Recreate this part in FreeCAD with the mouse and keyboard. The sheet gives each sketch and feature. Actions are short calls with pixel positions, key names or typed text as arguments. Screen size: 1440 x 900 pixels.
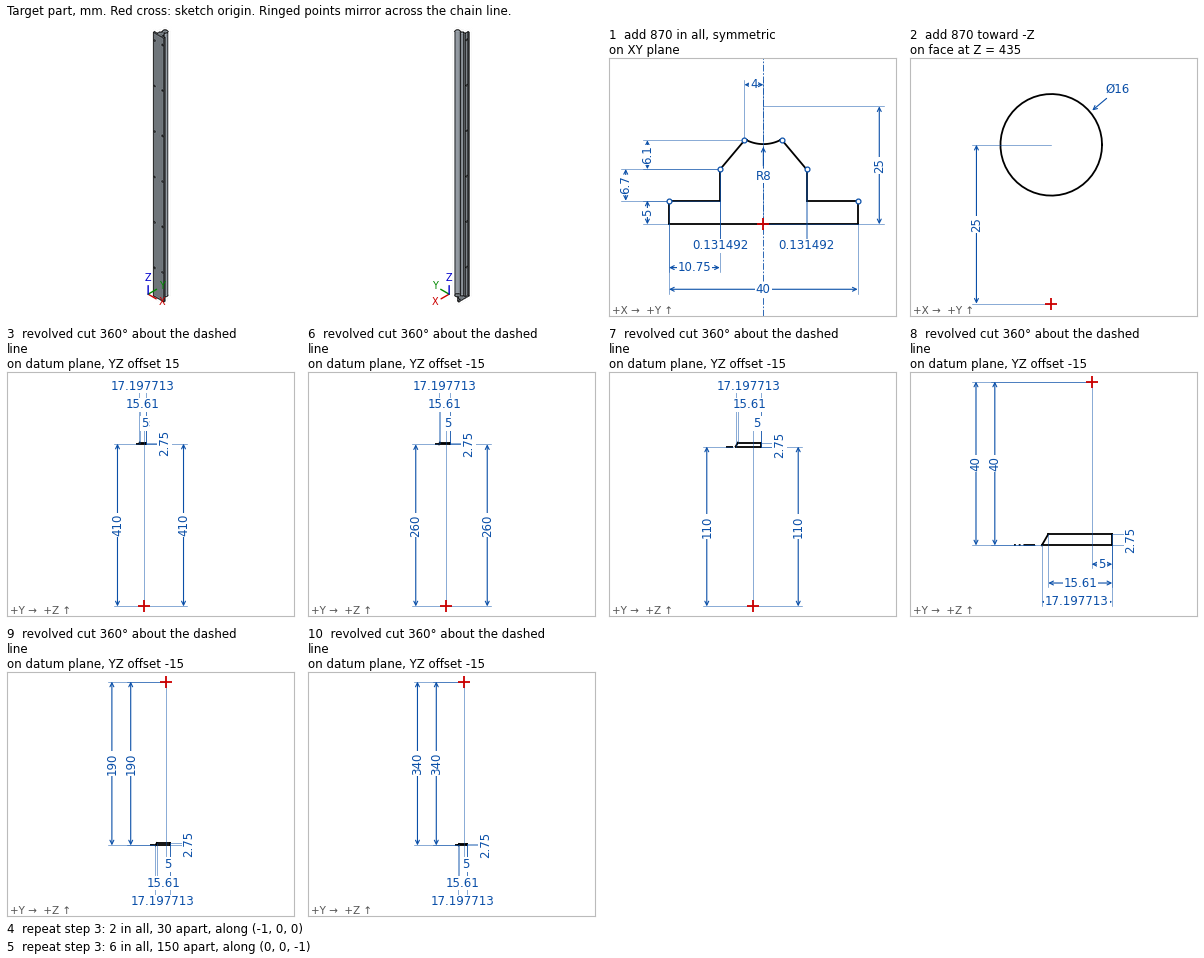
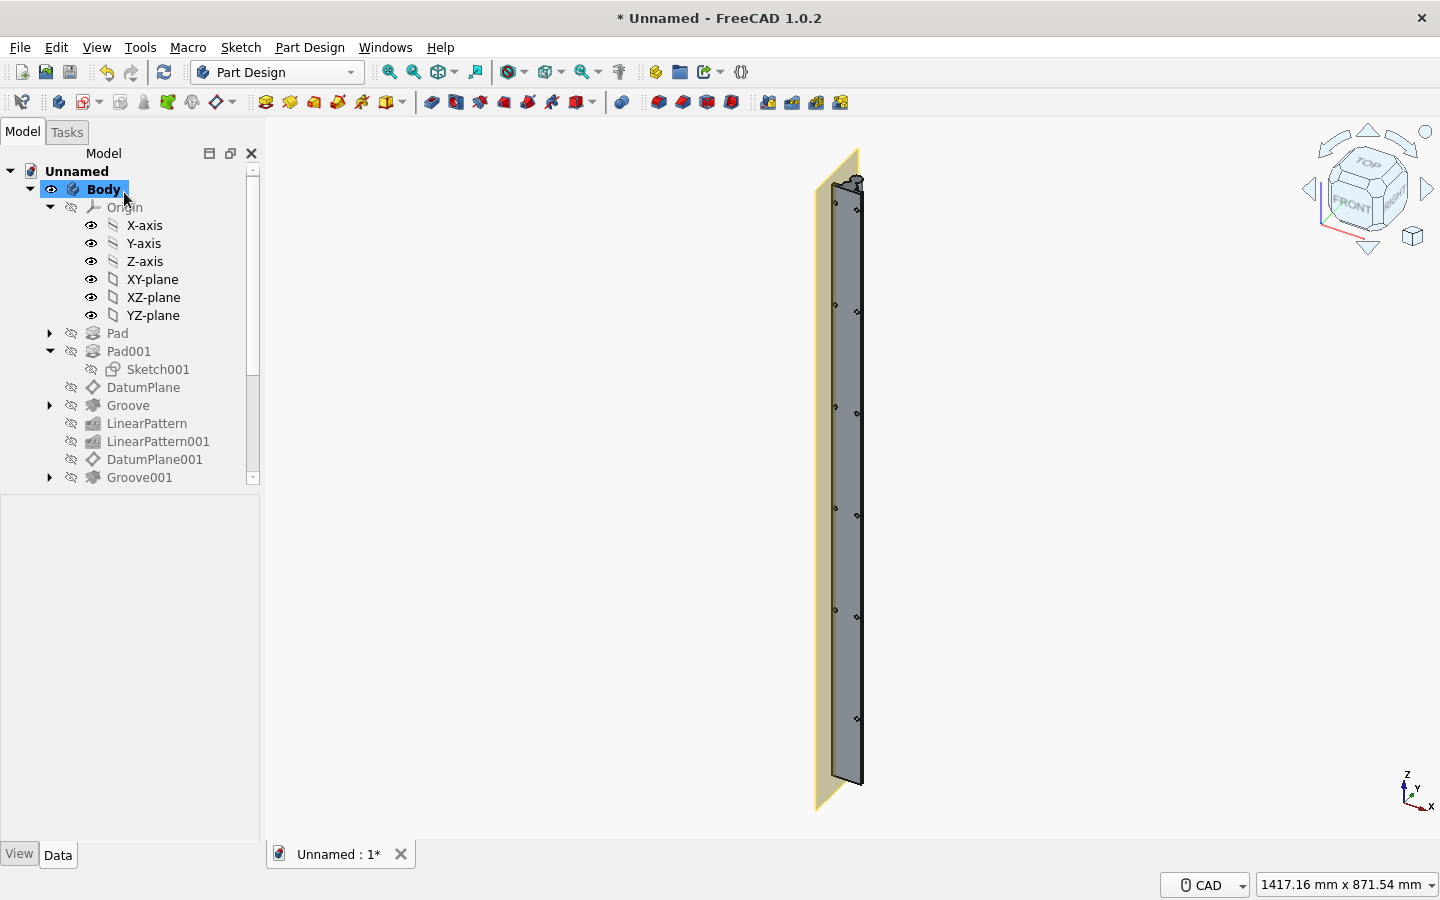
scroll(100, 329, down, 3)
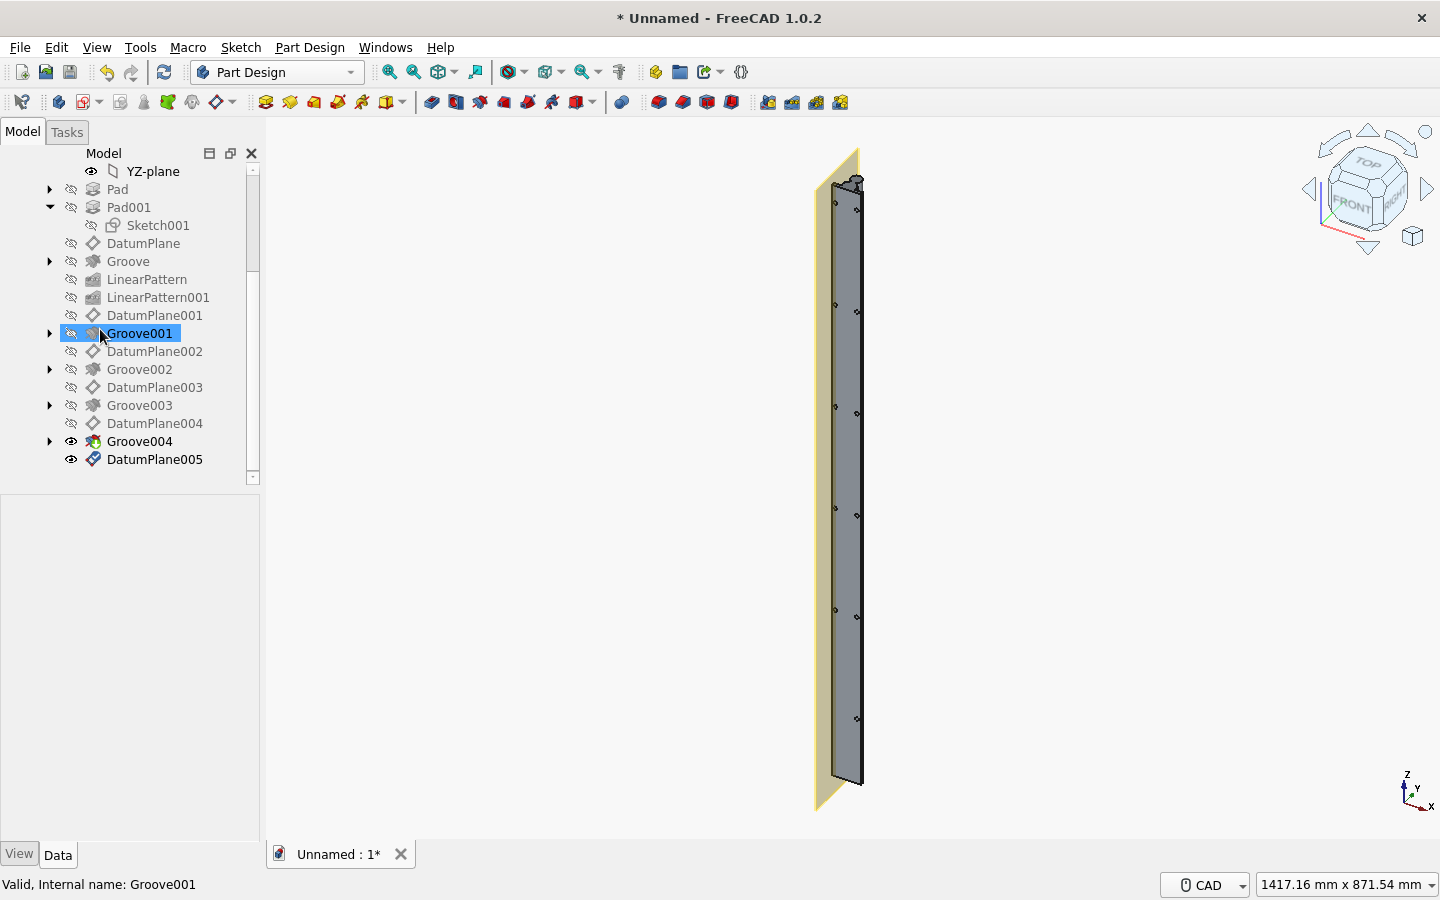
click(116, 459)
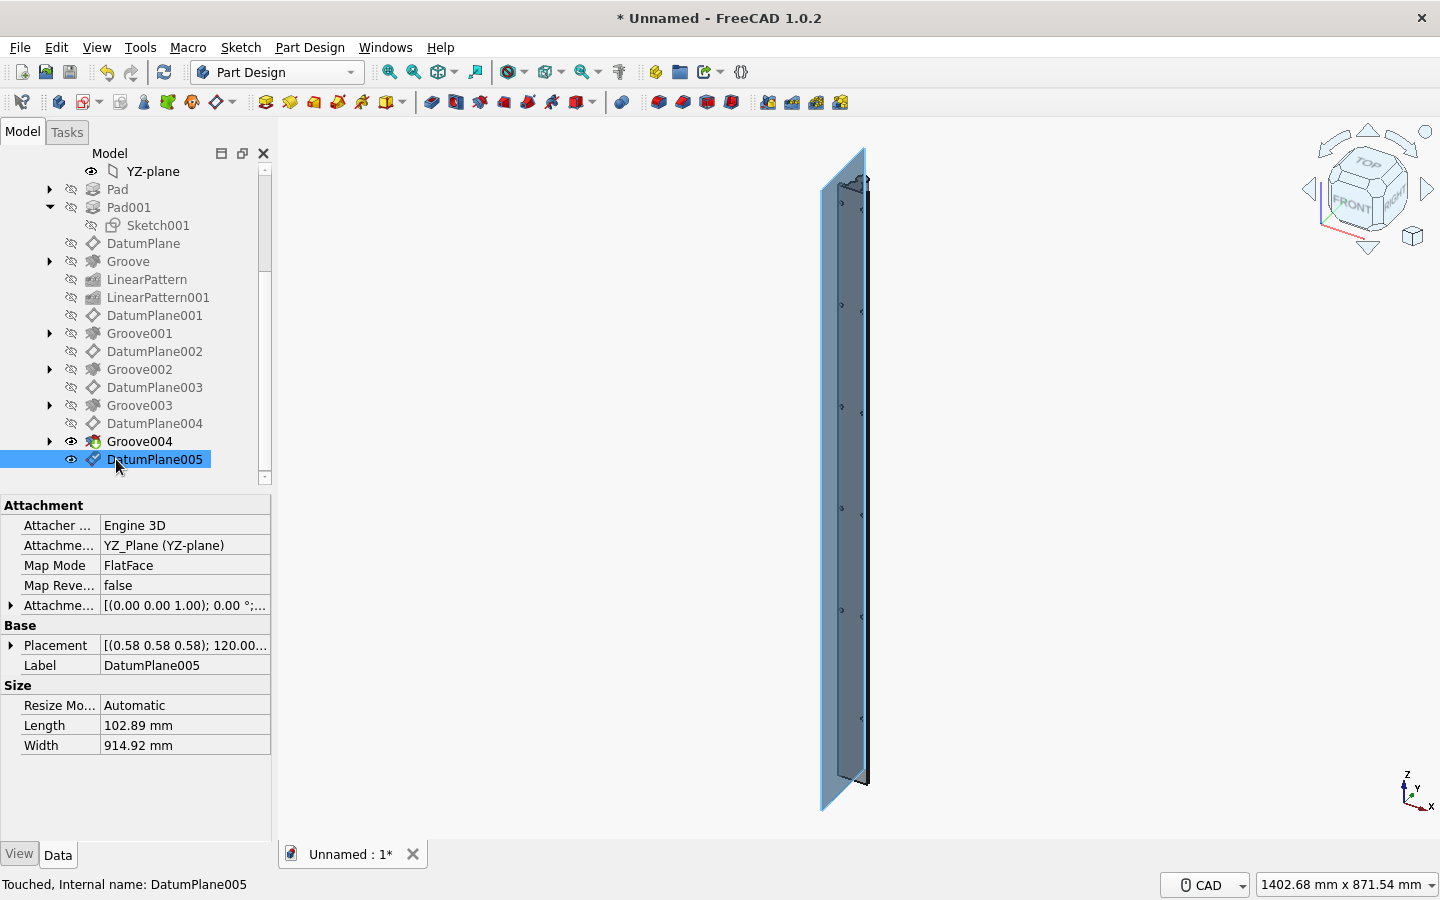
click(84, 102)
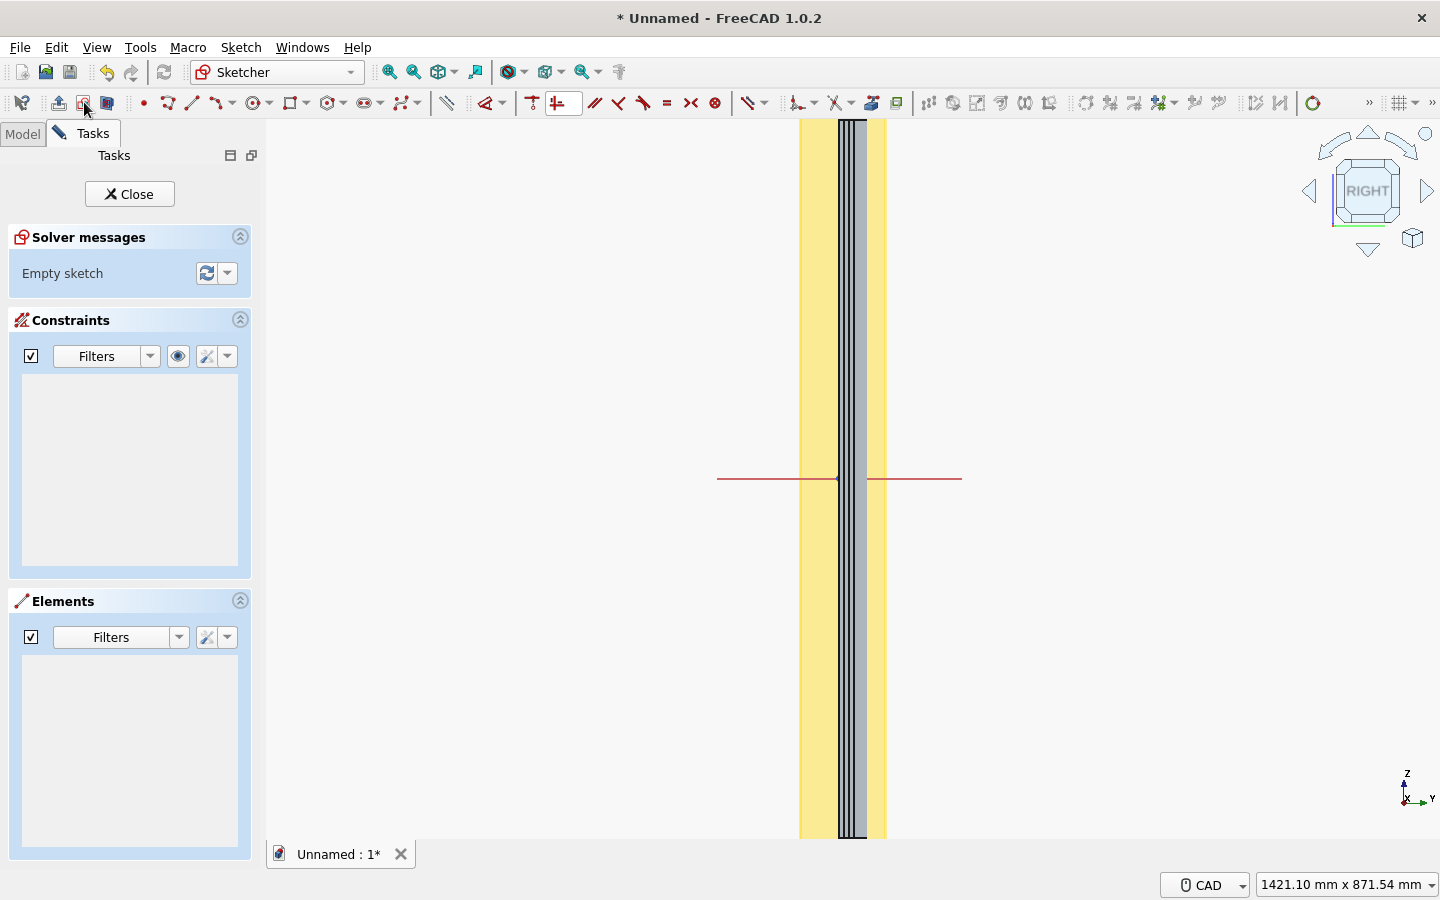
click(108, 104)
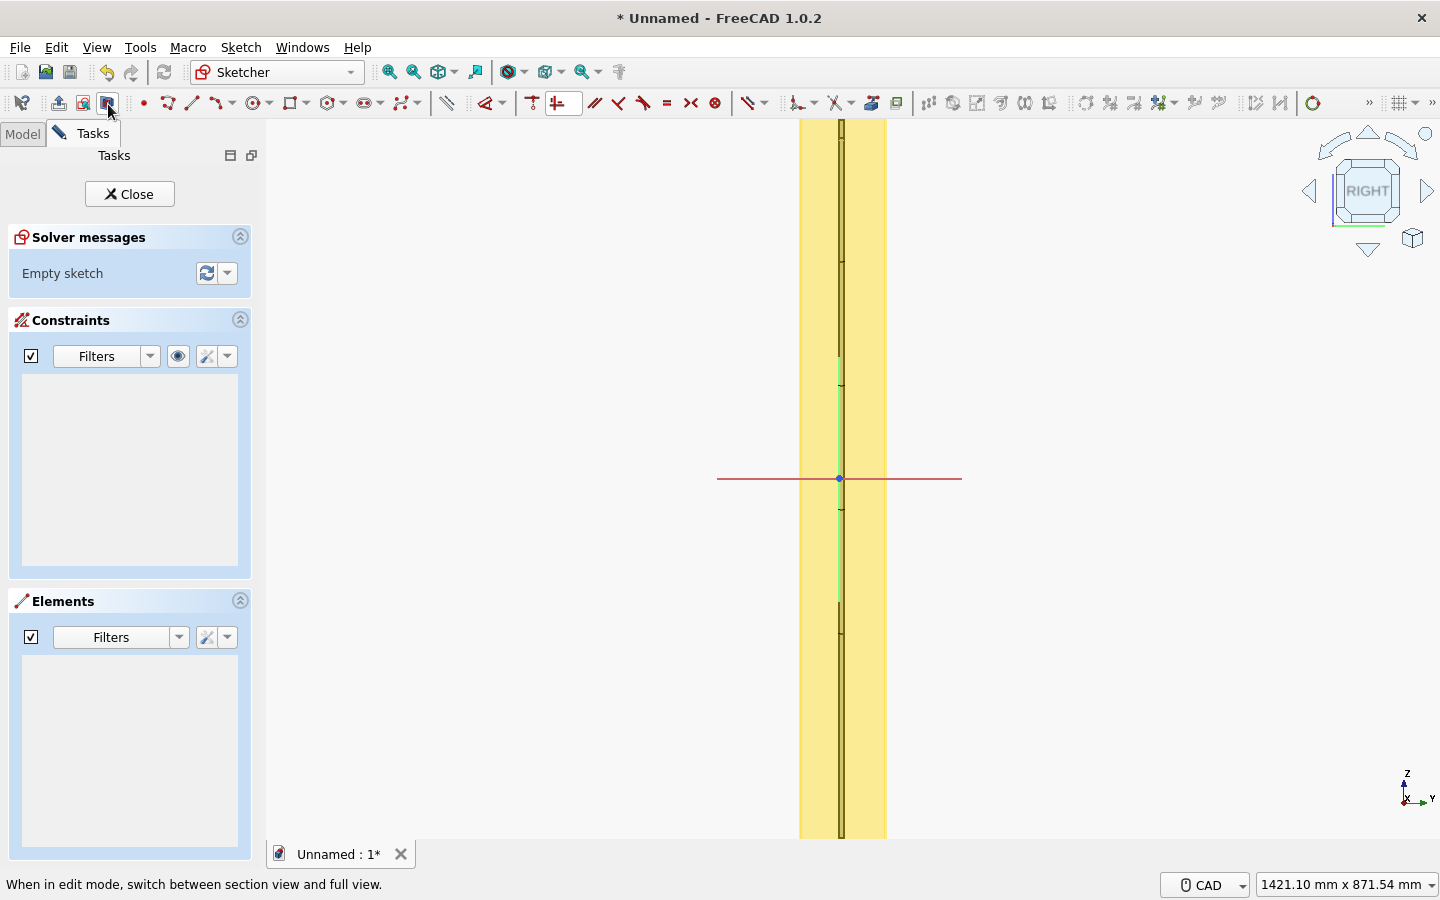
scroll(836, 773, up, 15)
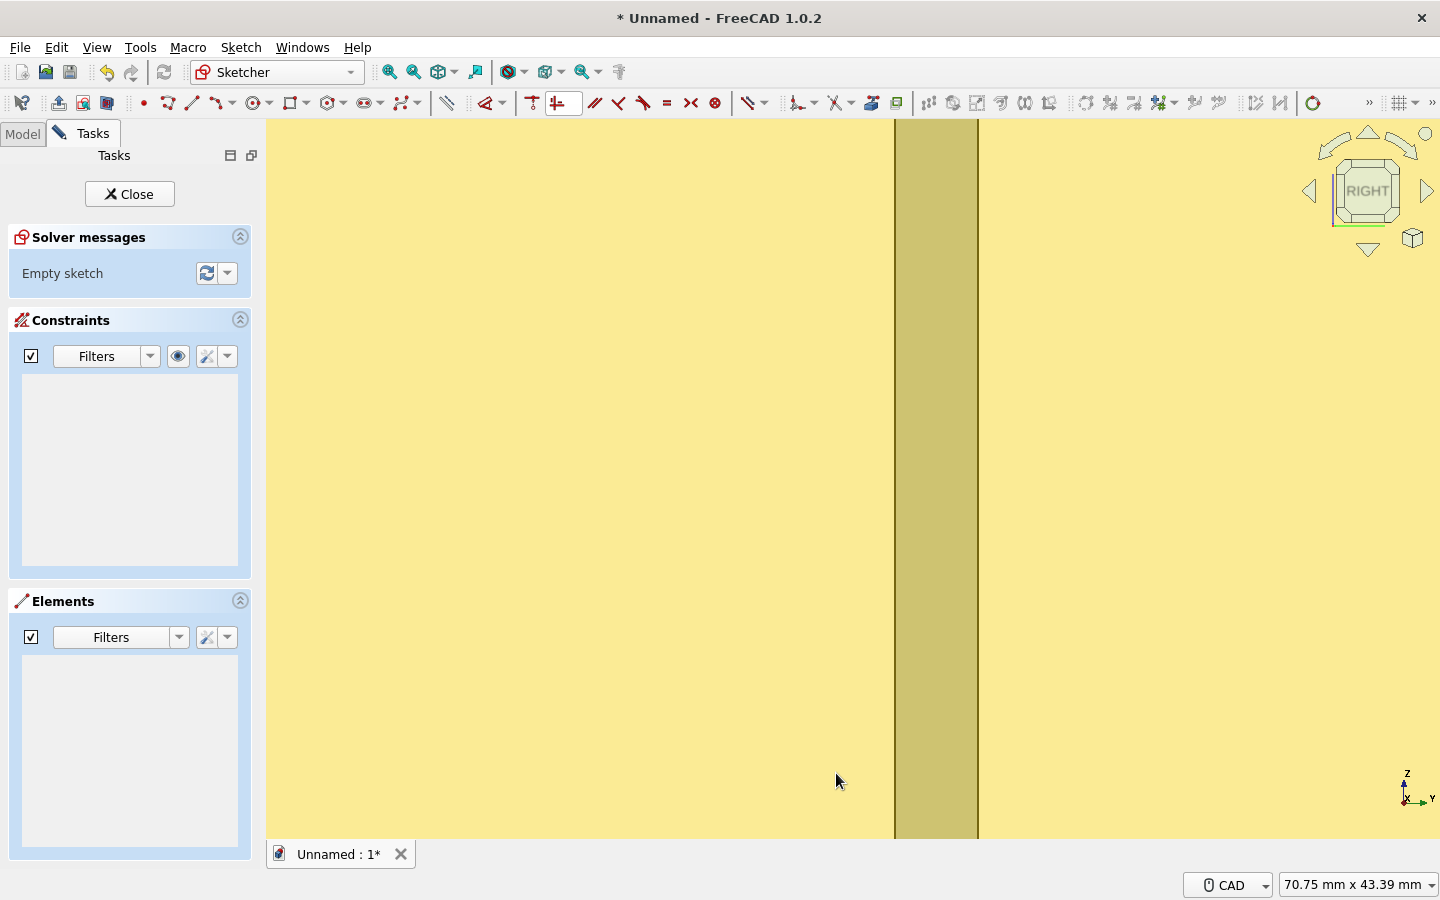
scroll(770, 458, up, 3)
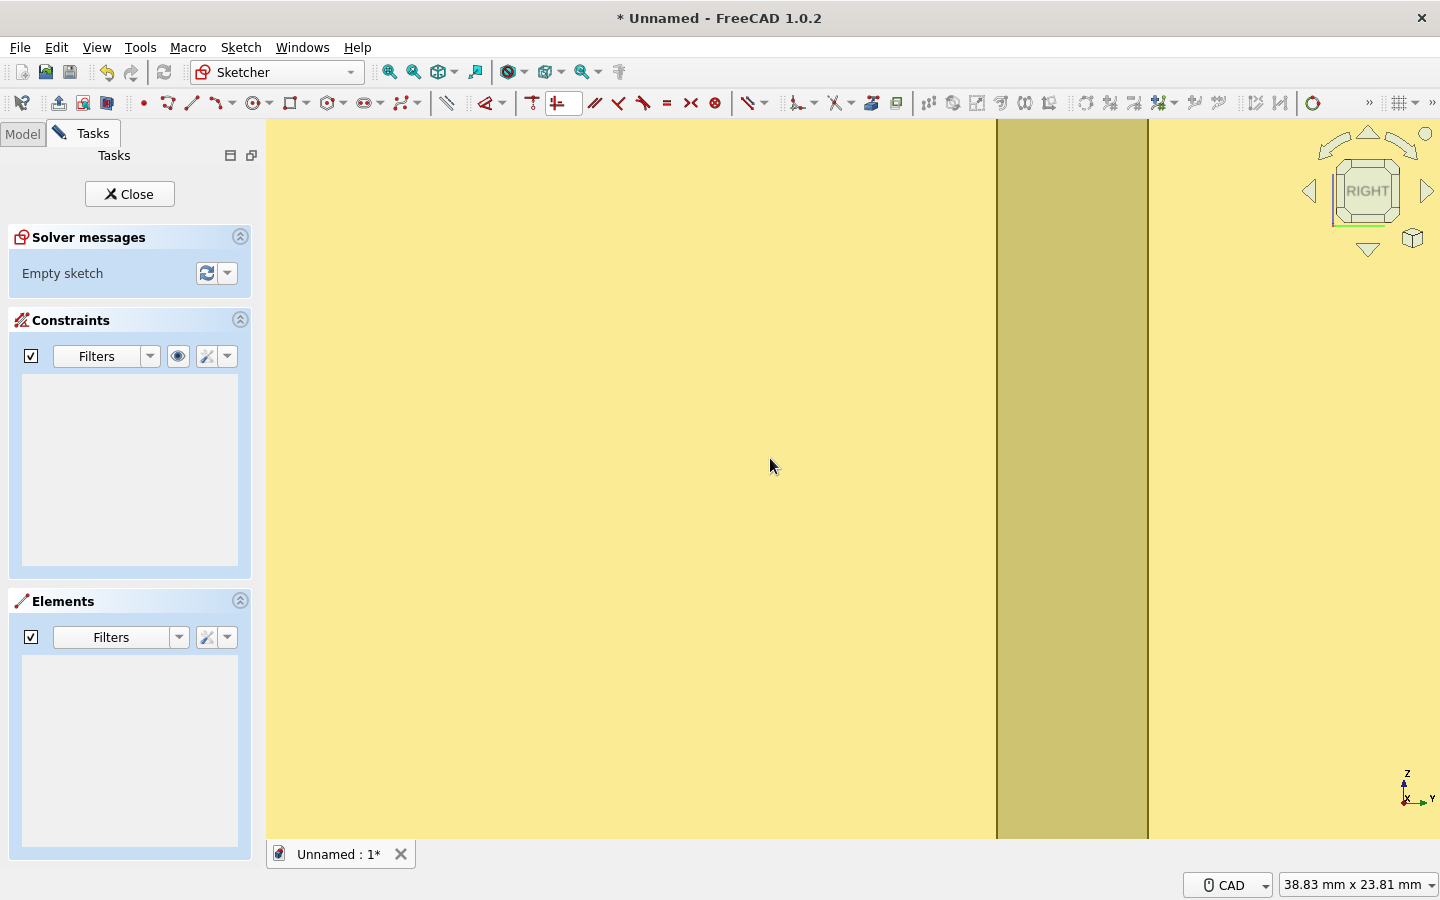
click(168, 104)